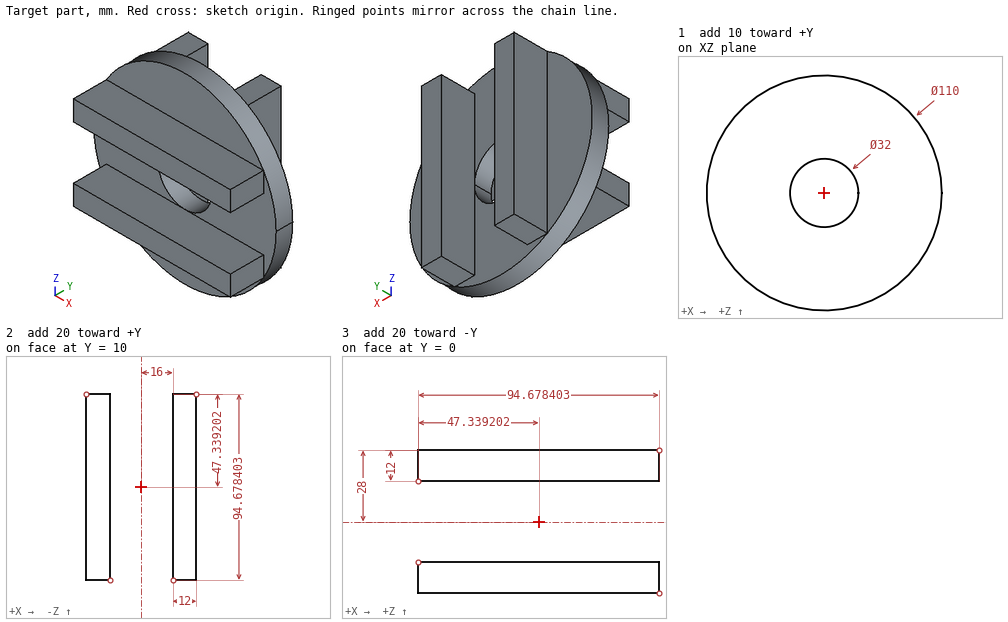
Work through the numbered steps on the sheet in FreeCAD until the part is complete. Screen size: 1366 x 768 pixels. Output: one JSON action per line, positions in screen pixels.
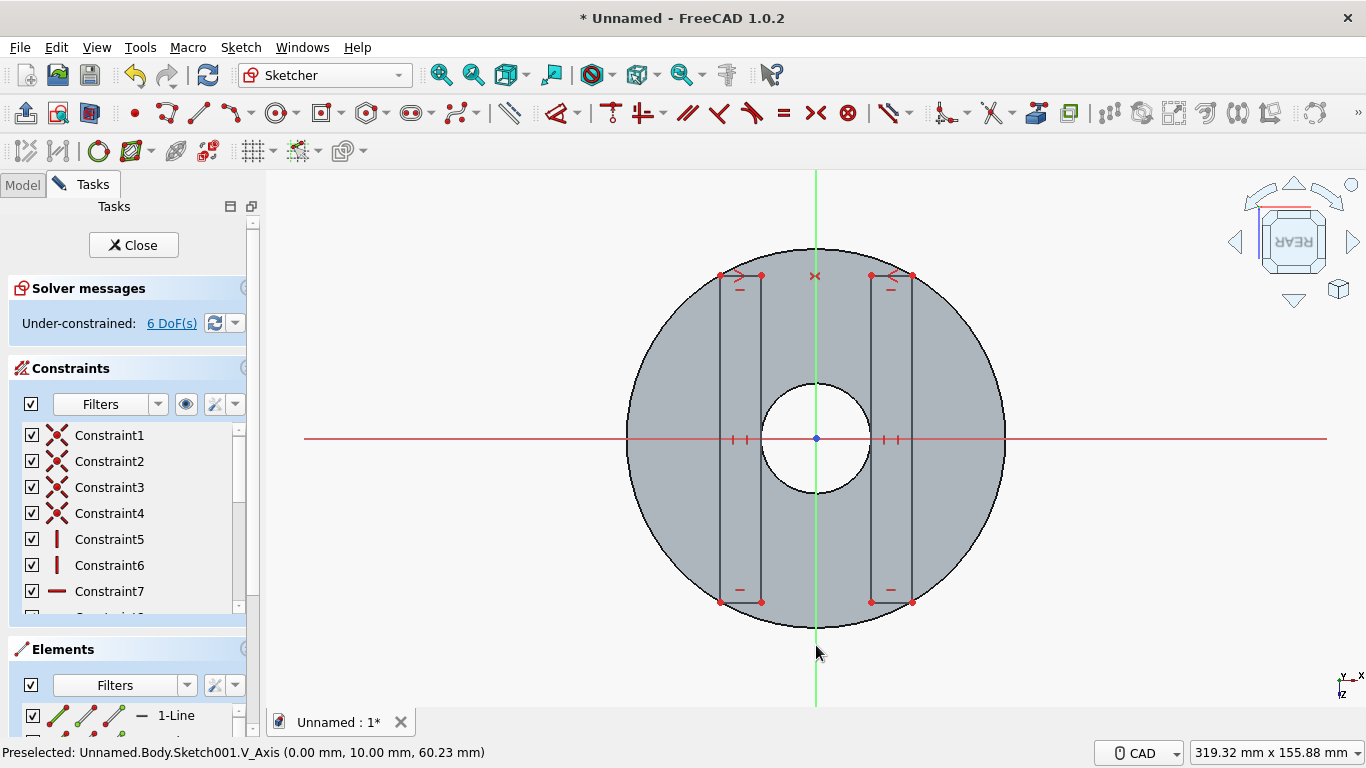
{"action": "left_click", "coordinate": [871, 603]}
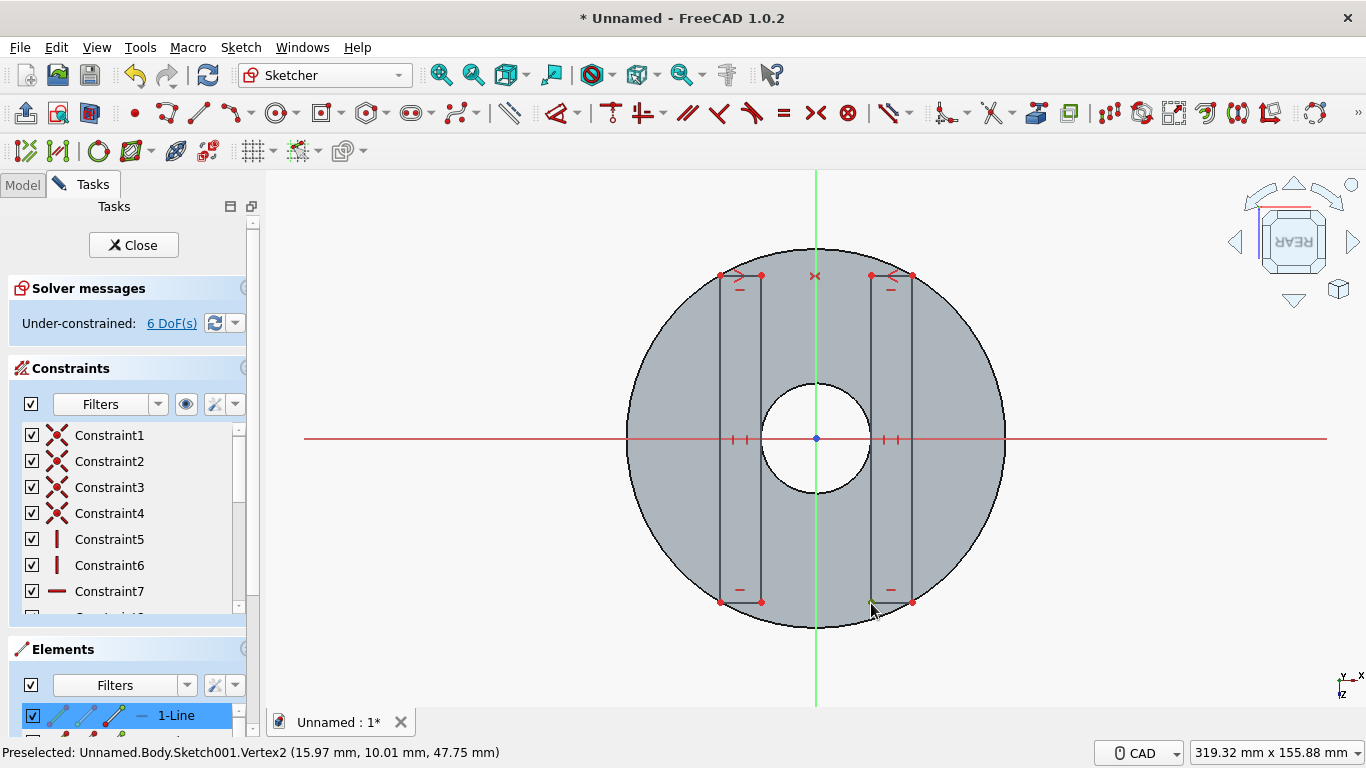
{"action": "left_click", "coordinate": [761, 603]}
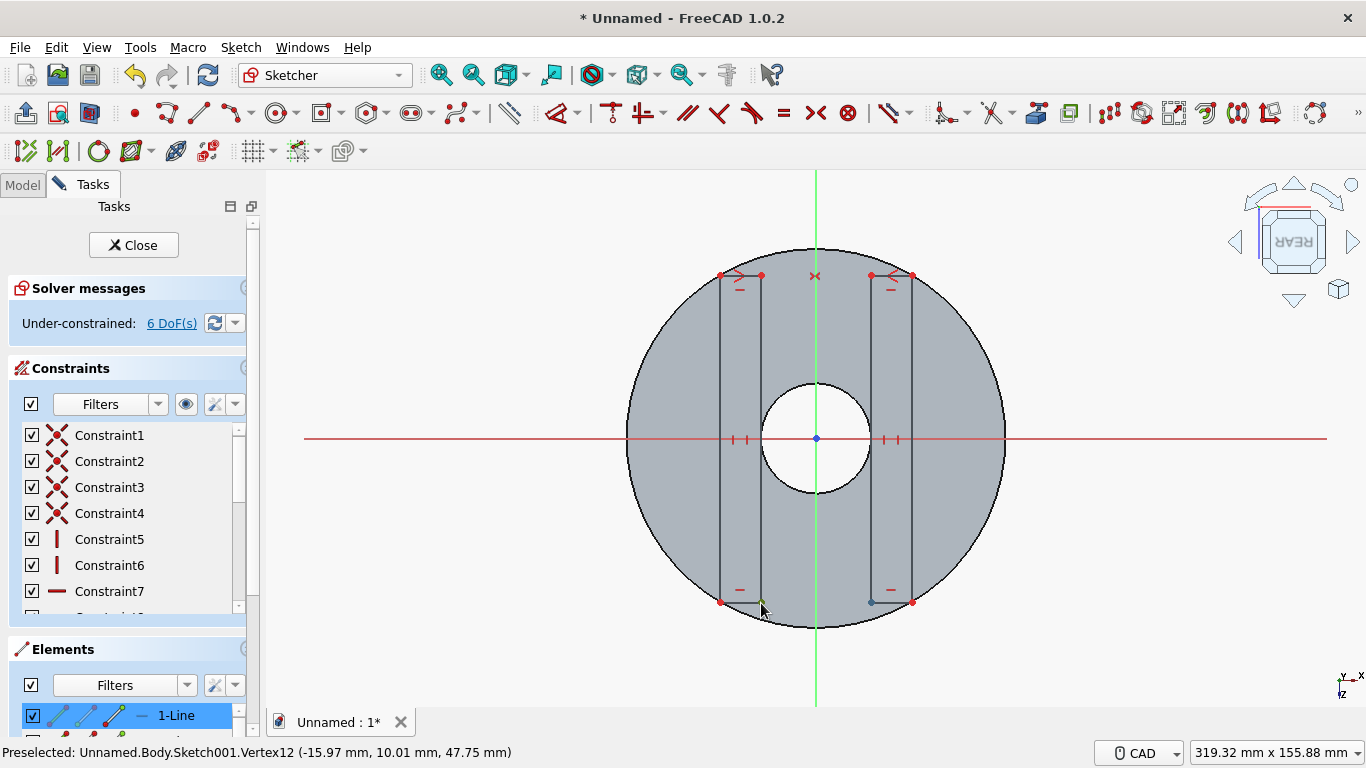
{"action": "left_click", "coordinate": [816, 645]}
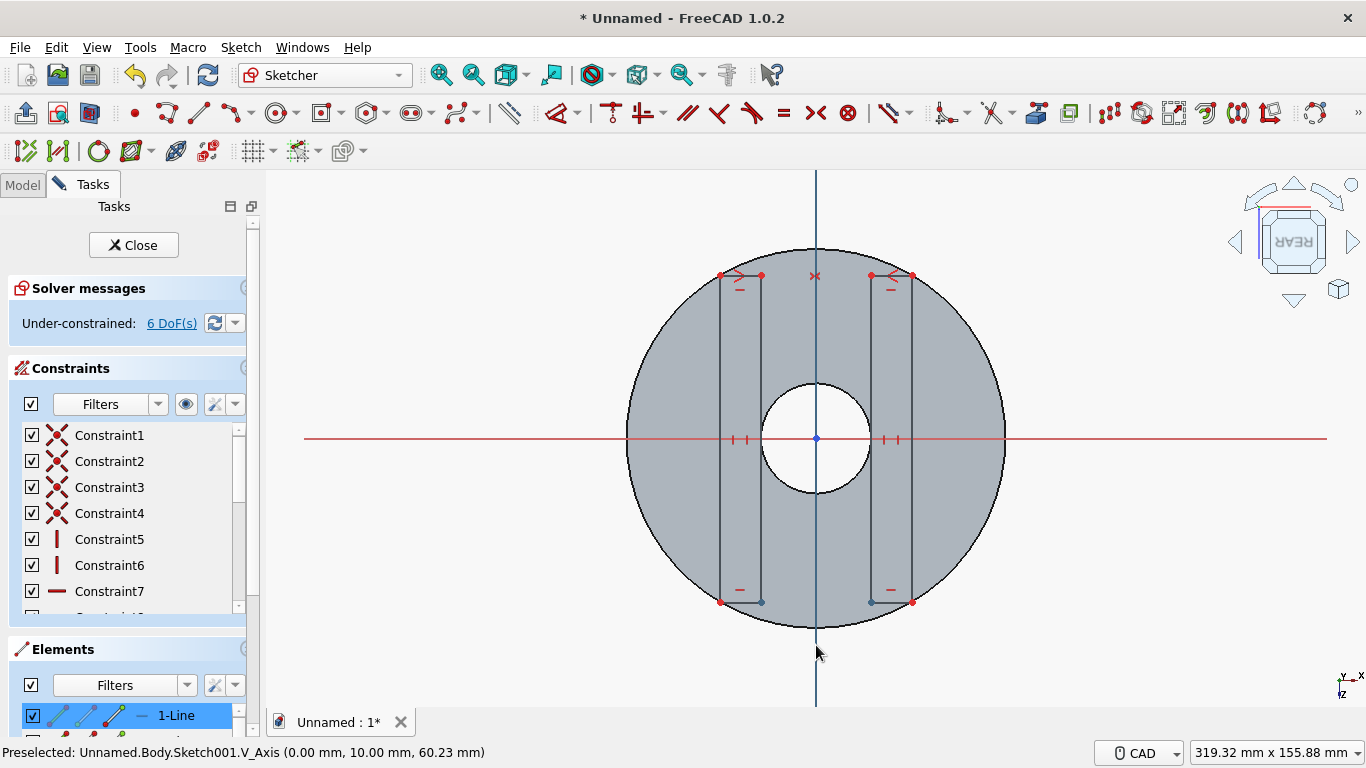
{"action": "key", "text": "s"}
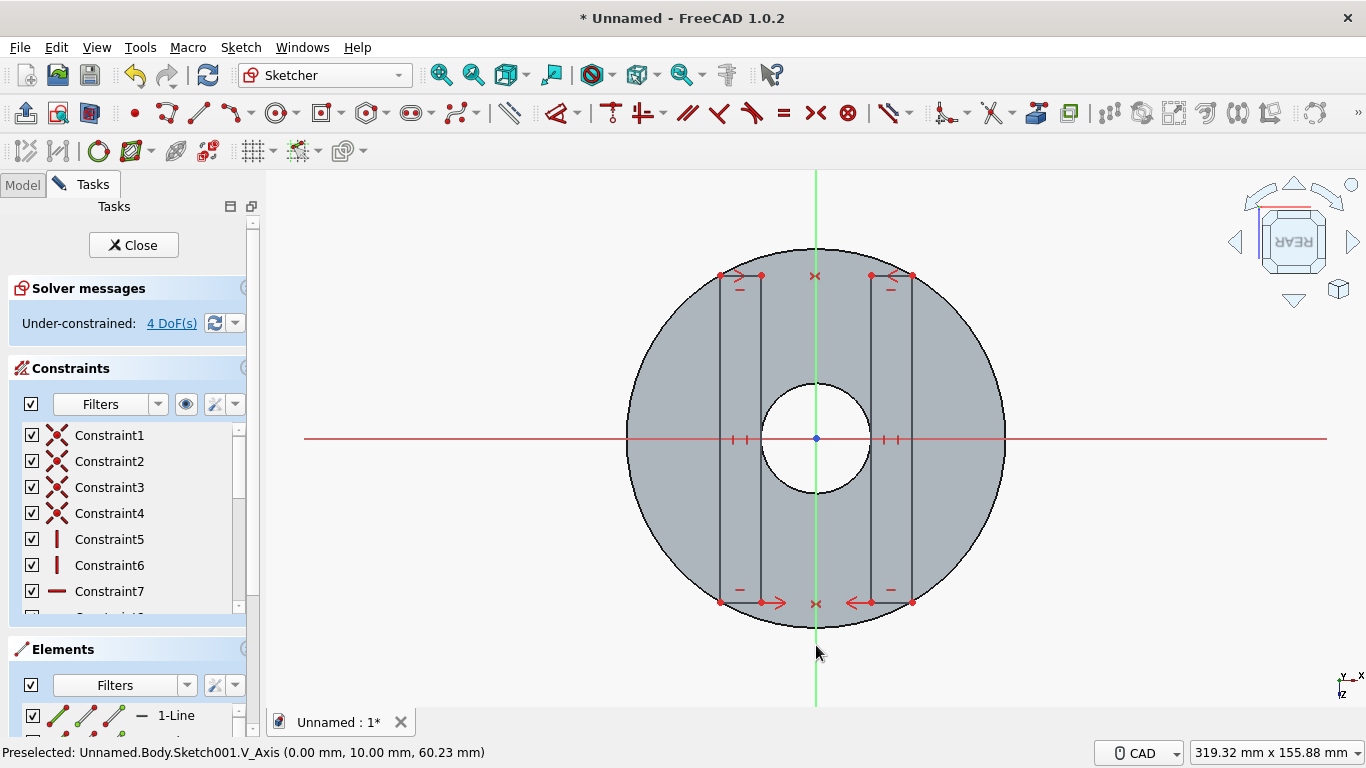
{"action": "left_click", "coordinate": [883, 603]}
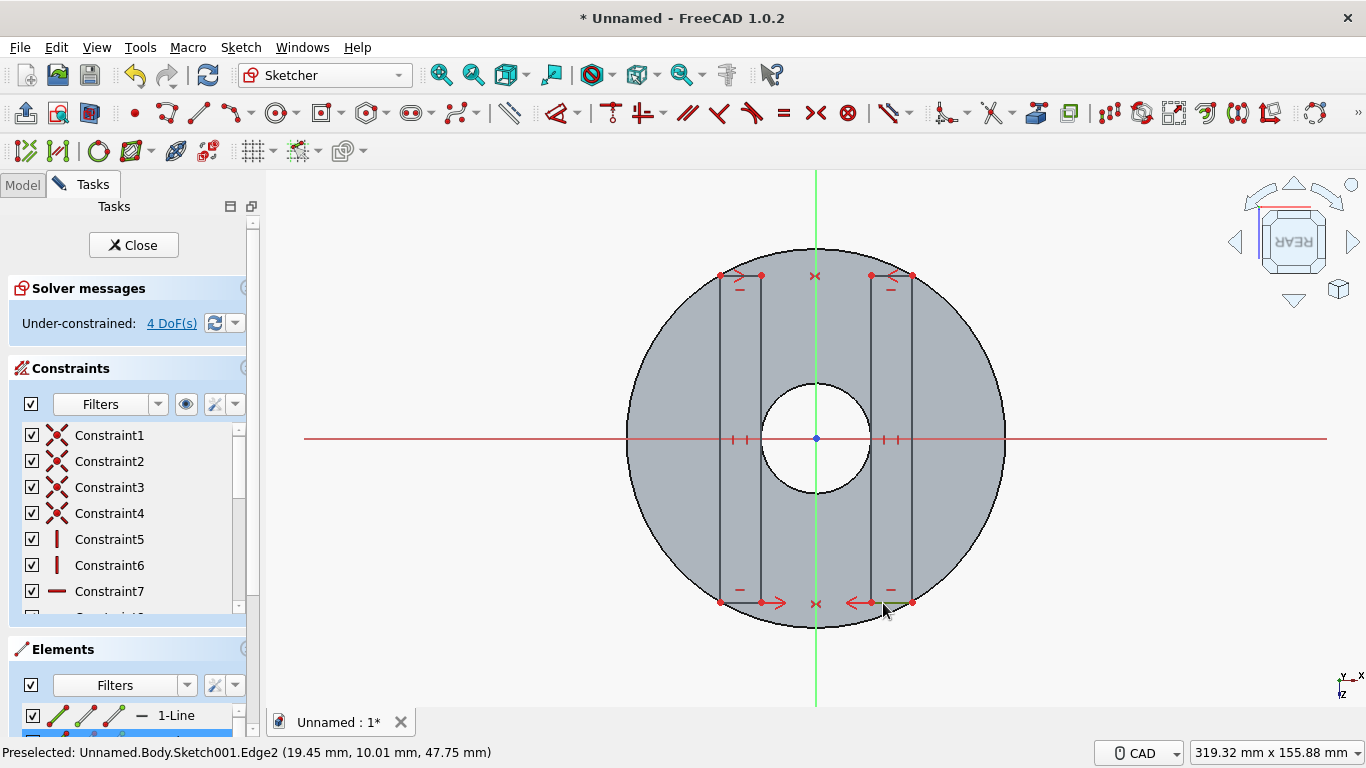
{"action": "key", "text": "l"}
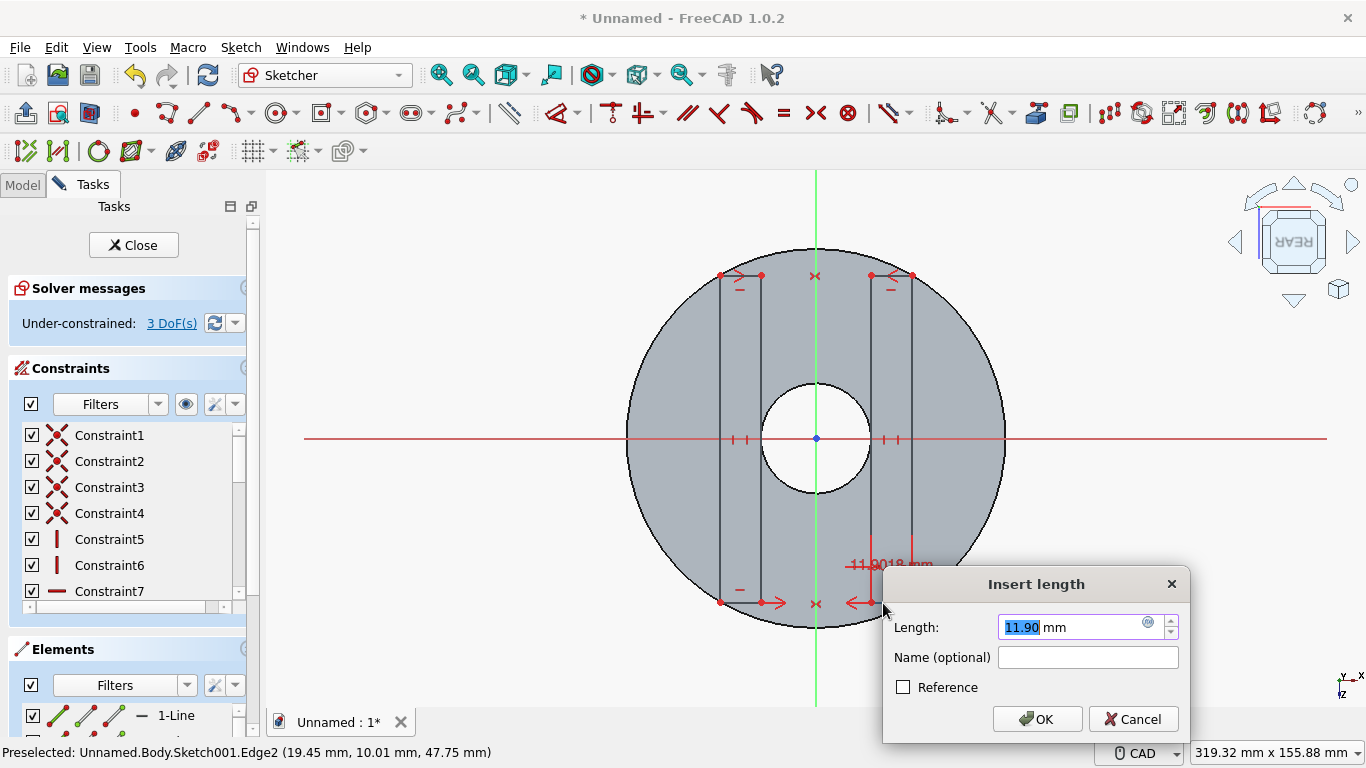
{"action": "type", "text": "12"}
{"action": "key", "text": "Return"}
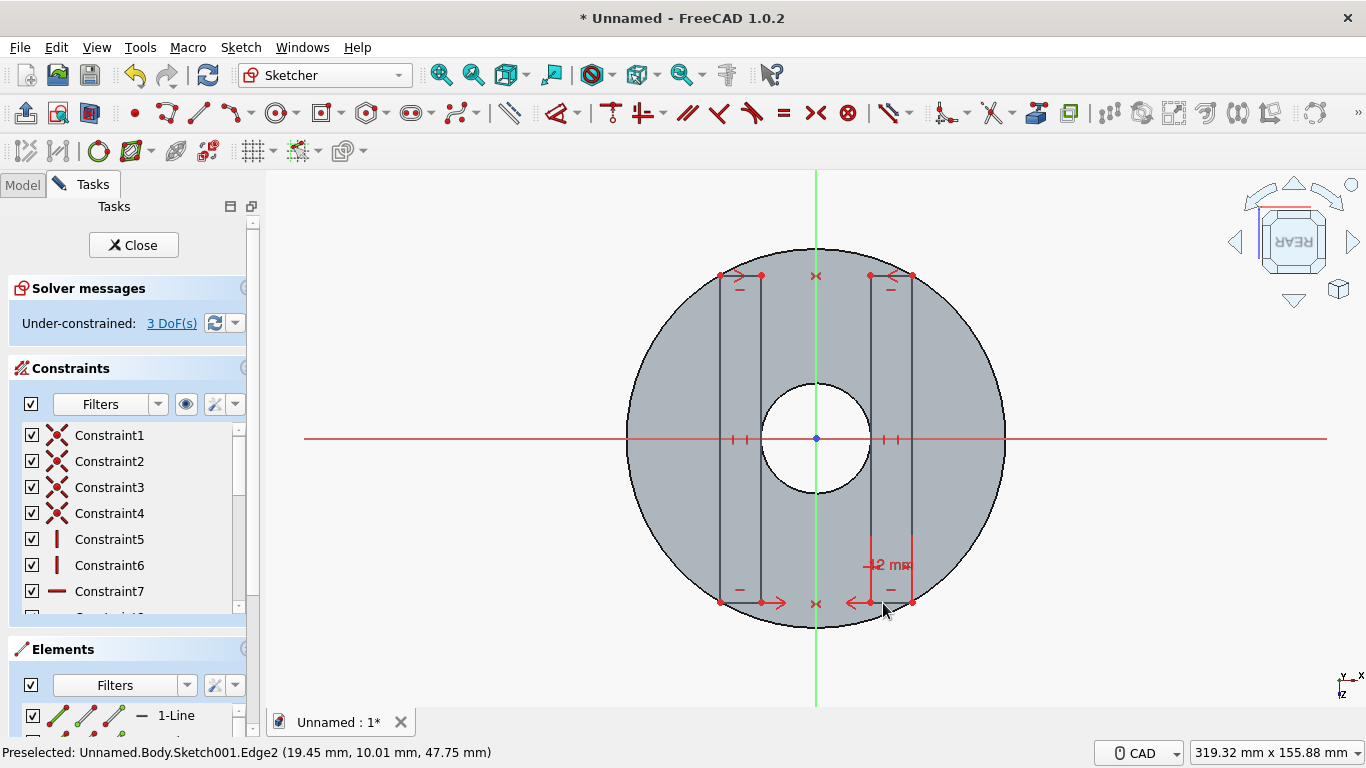
{"action": "left_click", "coordinate": [871, 276]}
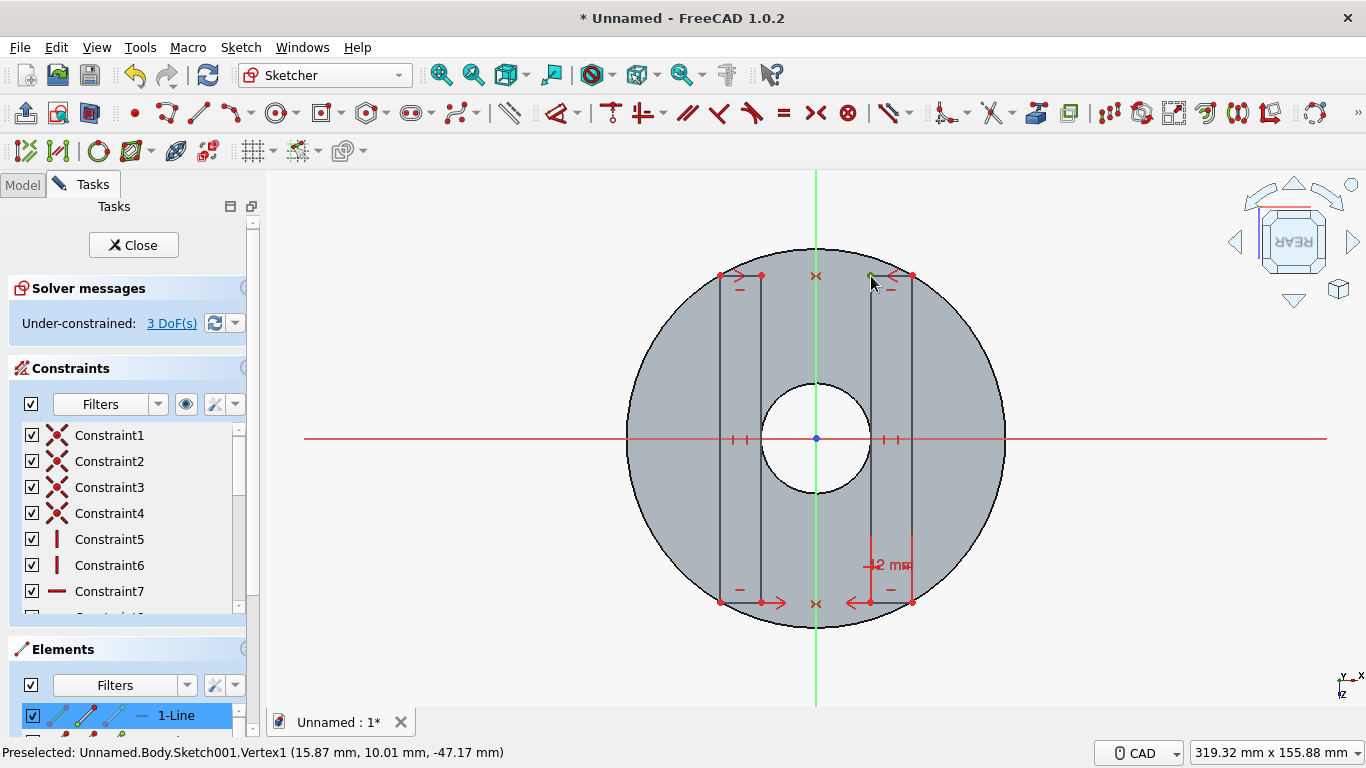
{"action": "key", "text": "l"}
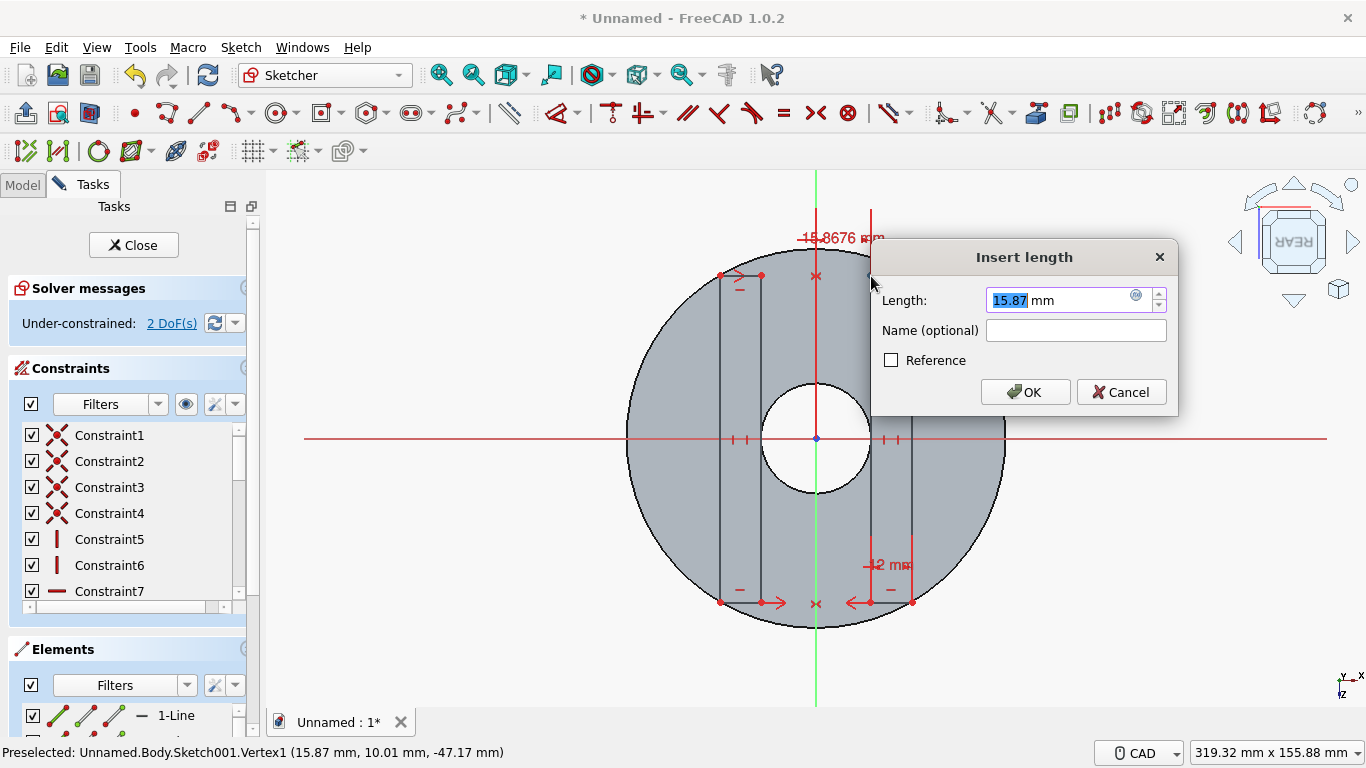
{"action": "type", "text": "16"}
{"action": "key", "text": "Return"}